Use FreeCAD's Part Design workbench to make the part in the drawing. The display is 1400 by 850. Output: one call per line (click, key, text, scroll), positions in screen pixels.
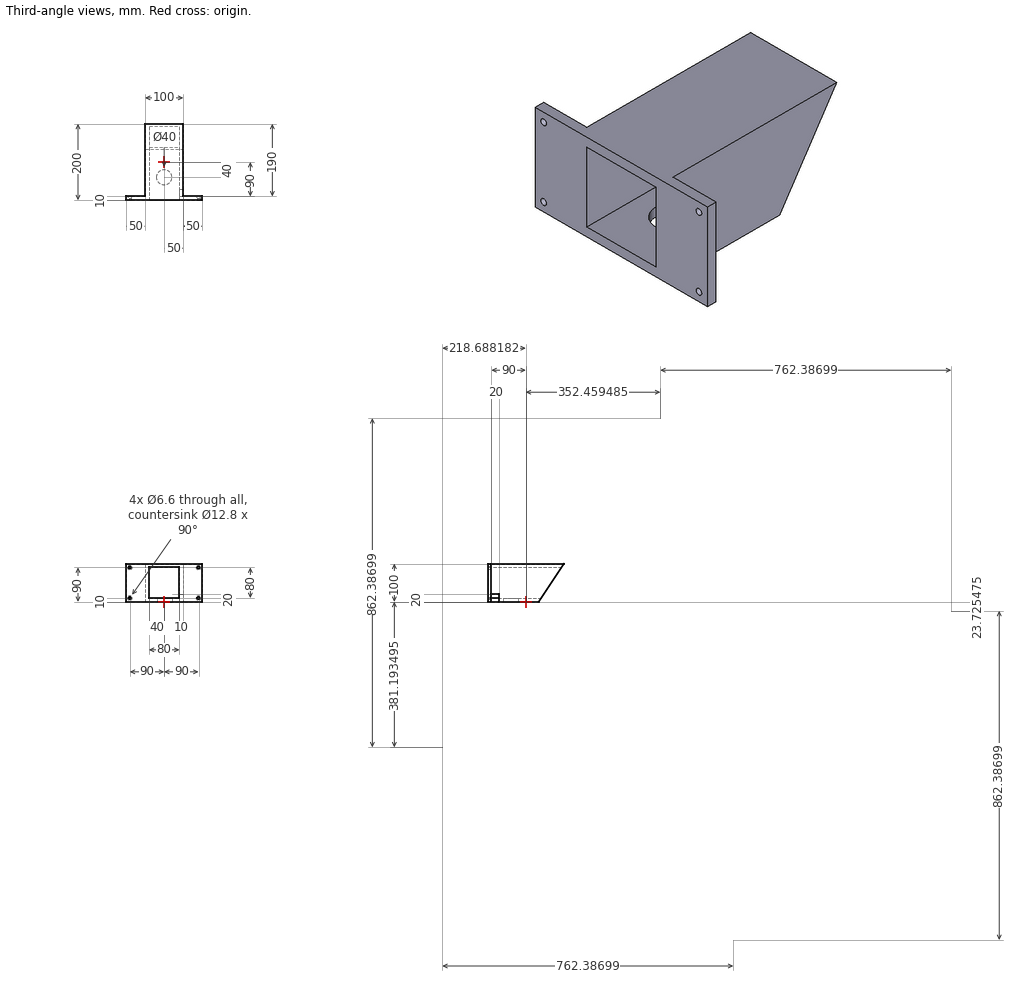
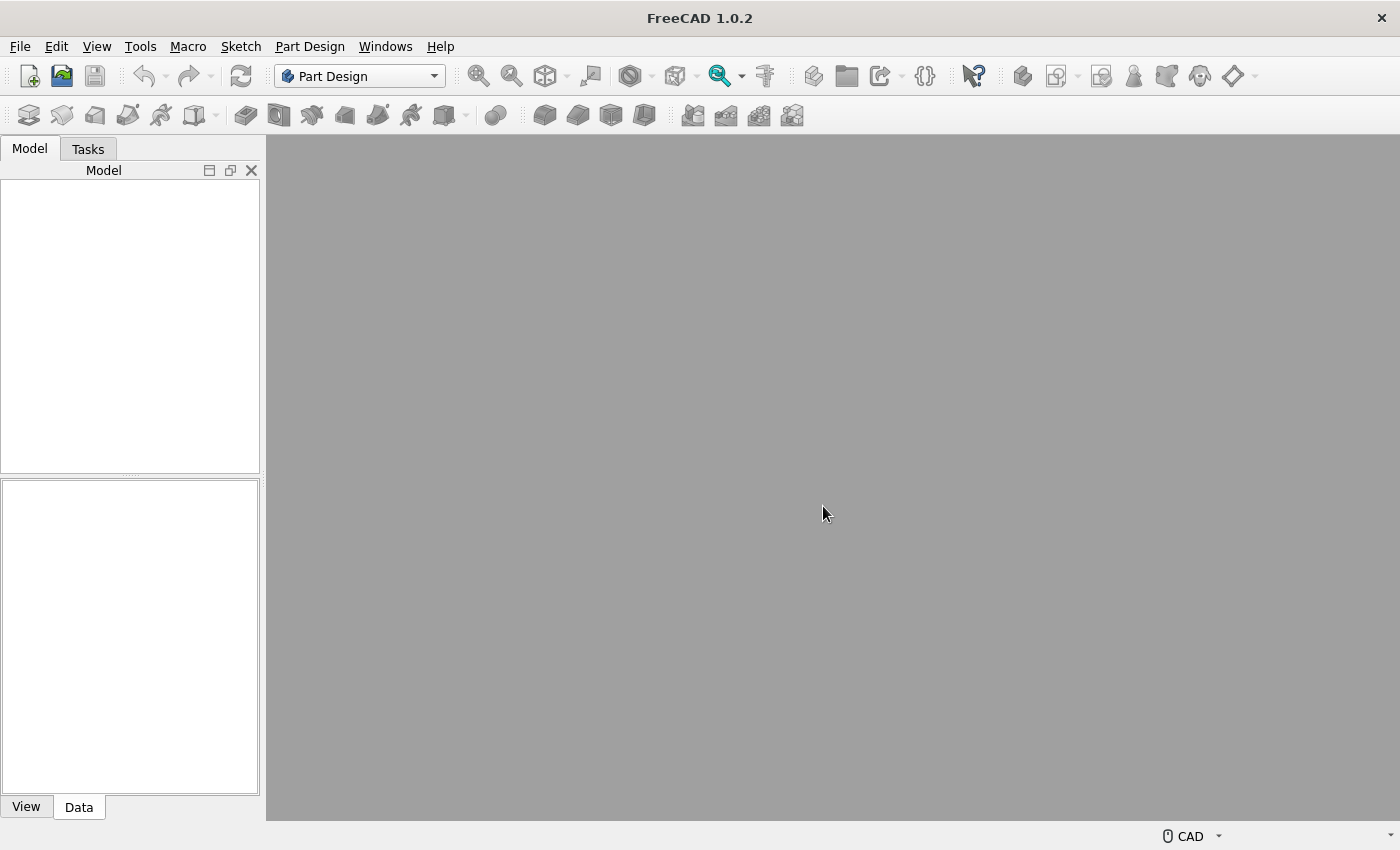
key(ctrl+n)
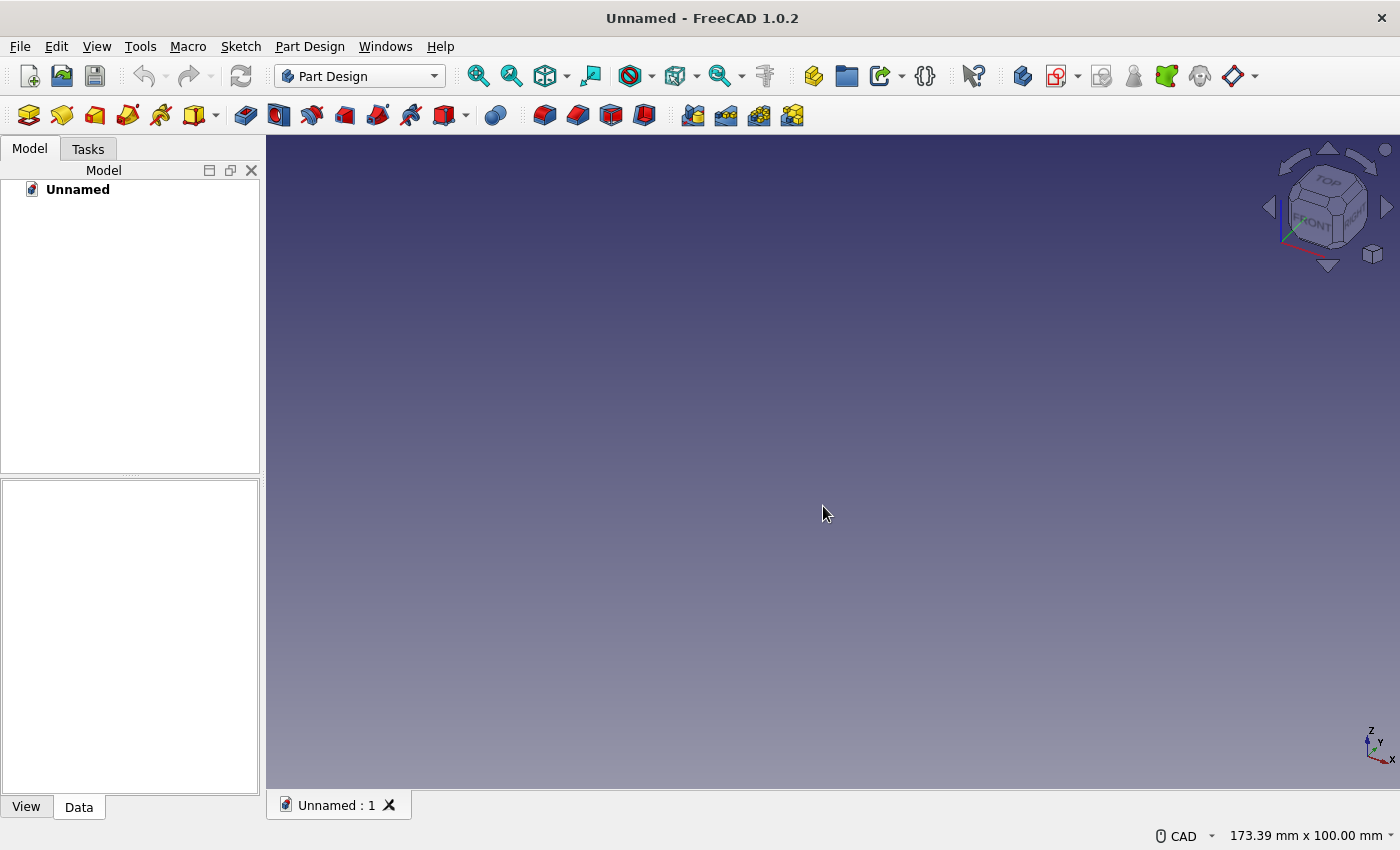
click(1056, 76)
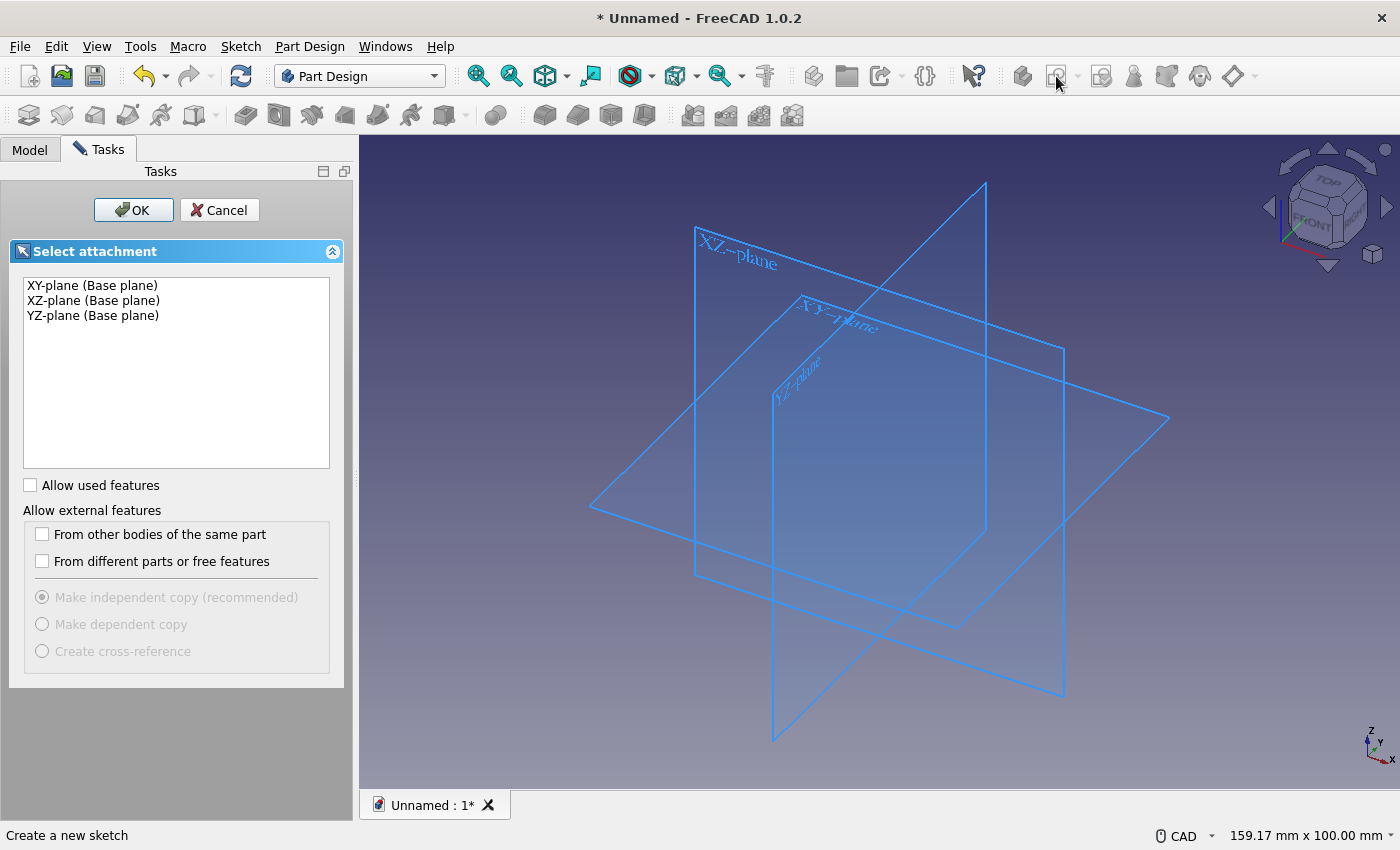
click(84, 286)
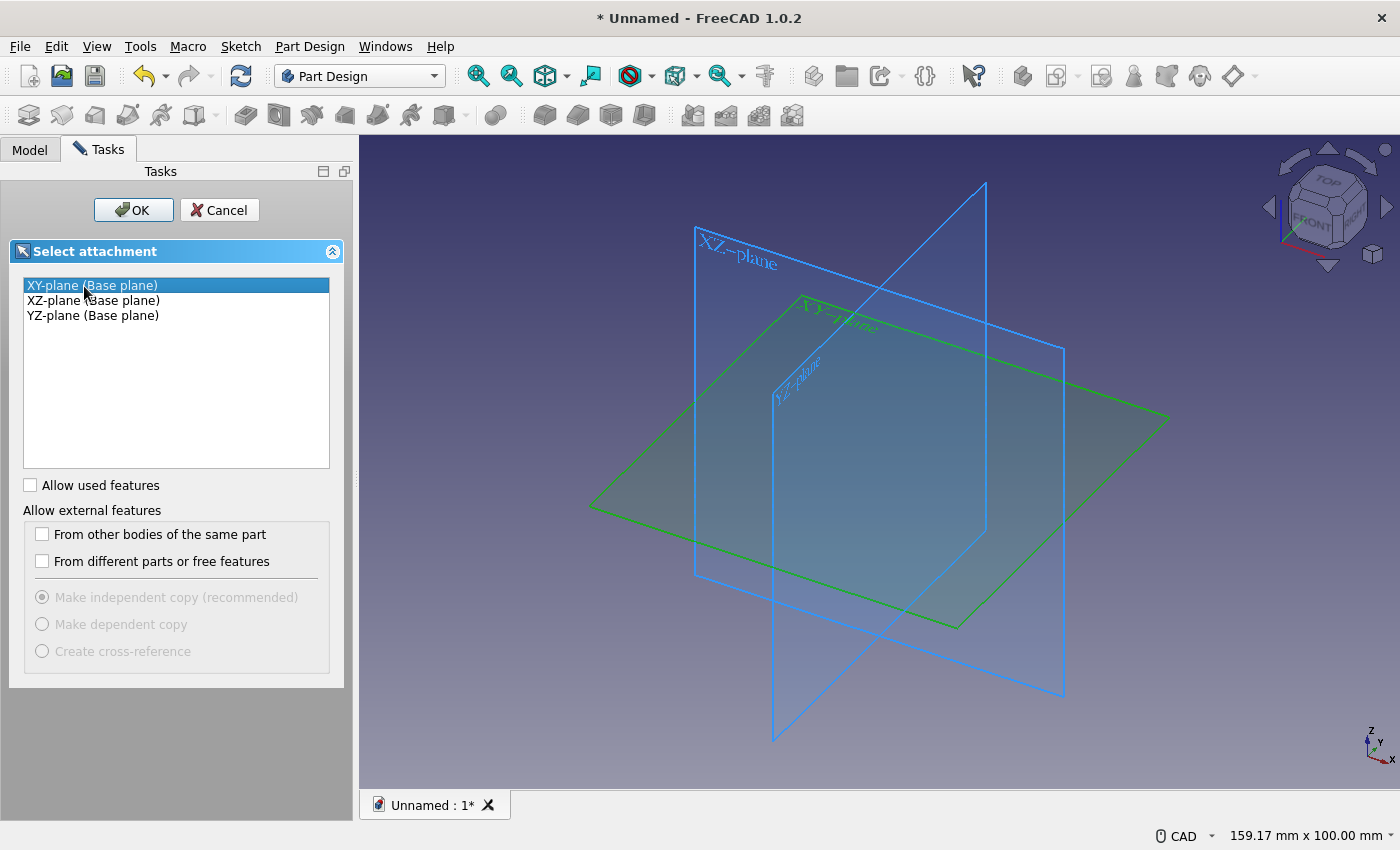
click(134, 210)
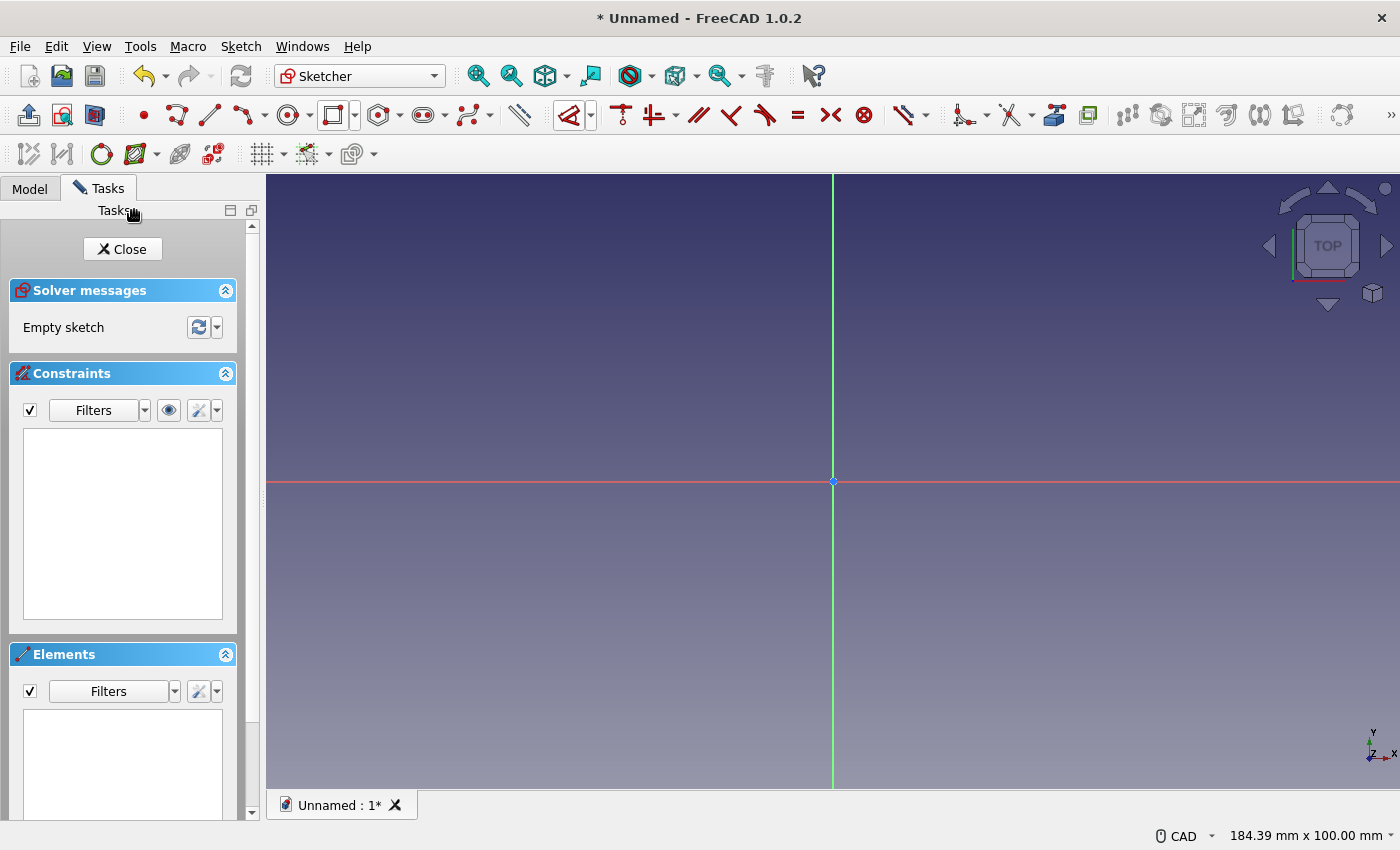
scroll(735, 482, down, 6)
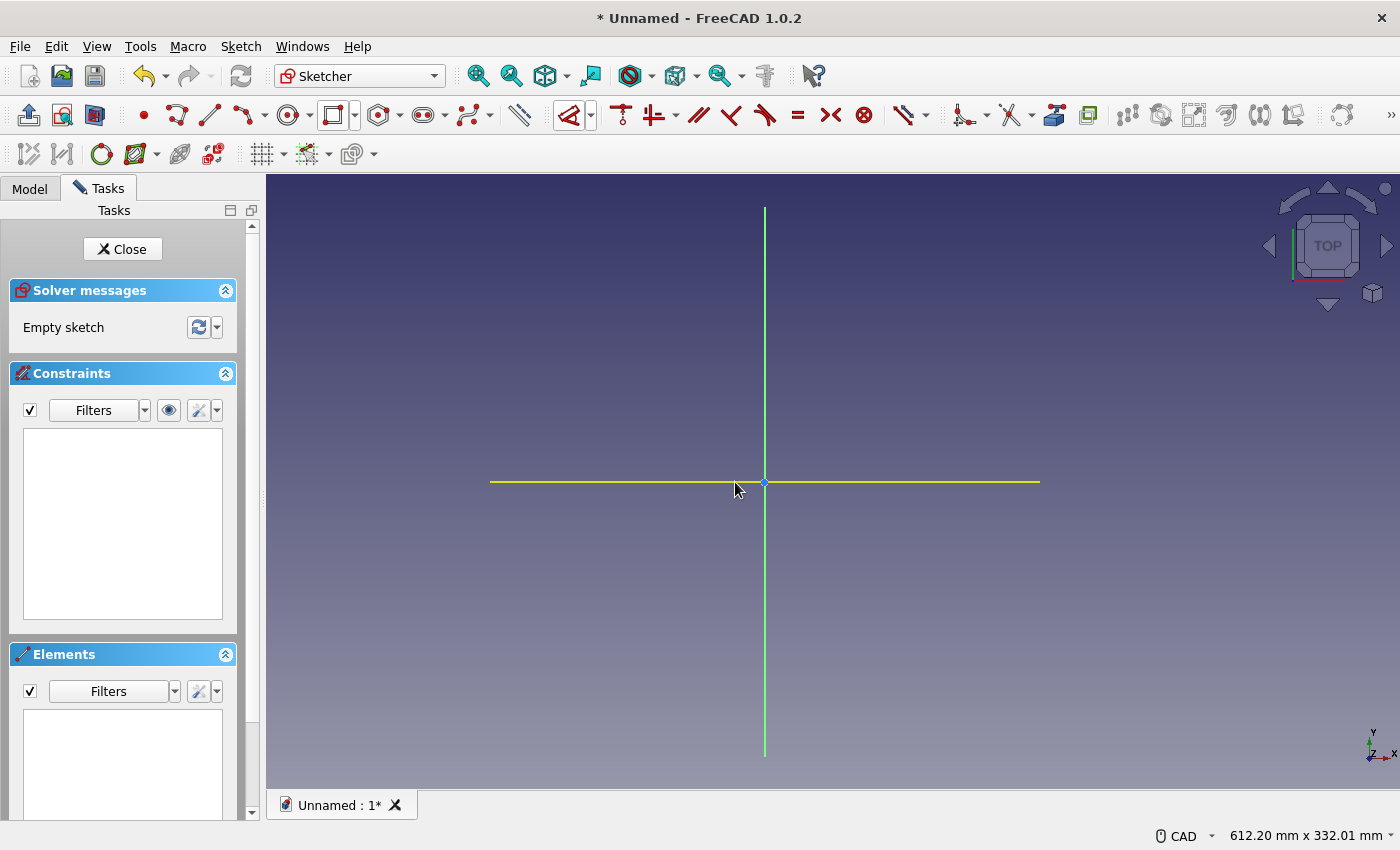
key(g)
key(m)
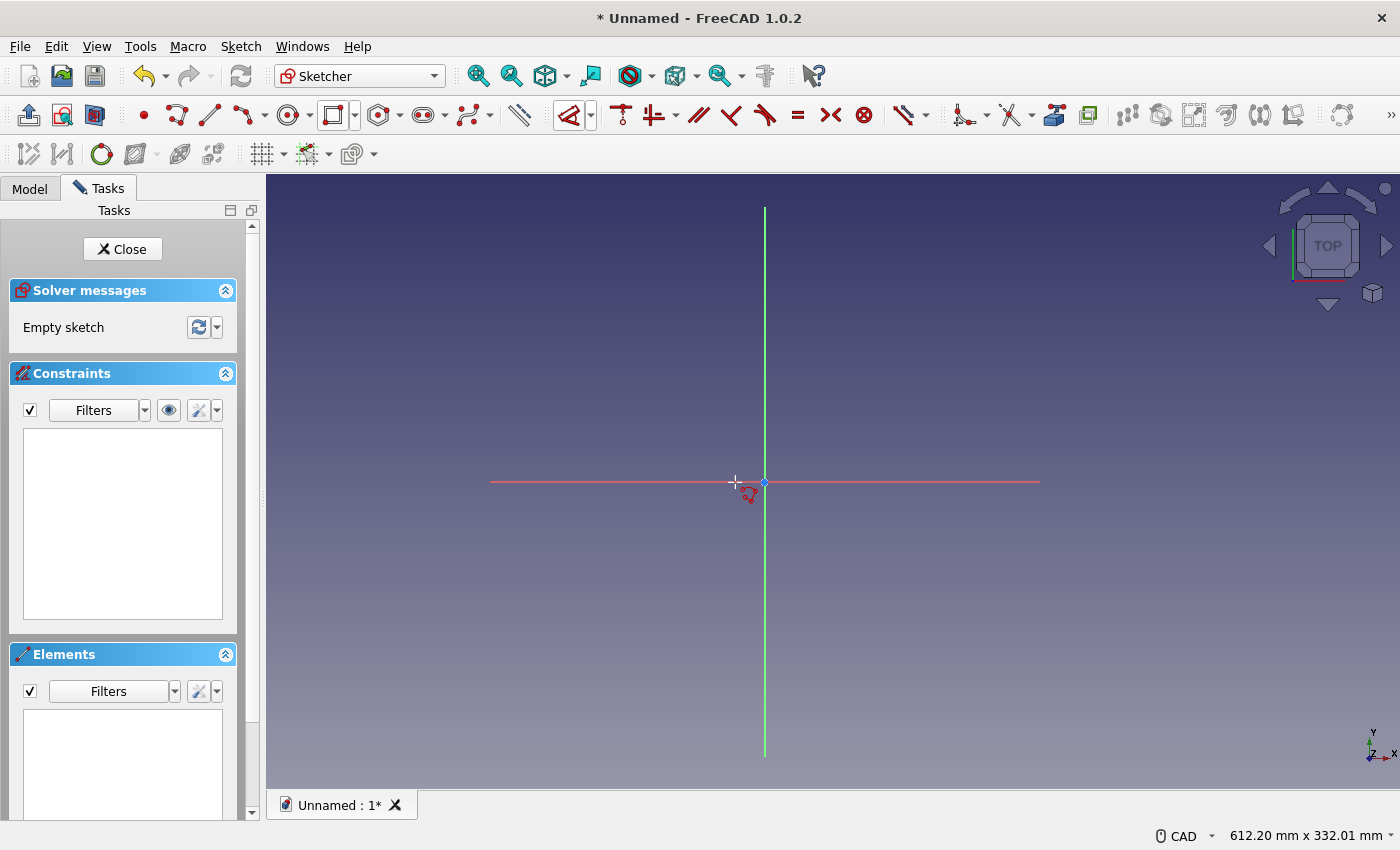
click(857, 649)
click(857, 297)
click(672, 297)
click(672, 649)
click(580, 649)
click(580, 667)
click(950, 667)
click(950, 649)
click(857, 650)
key(Escape)
key(Escape)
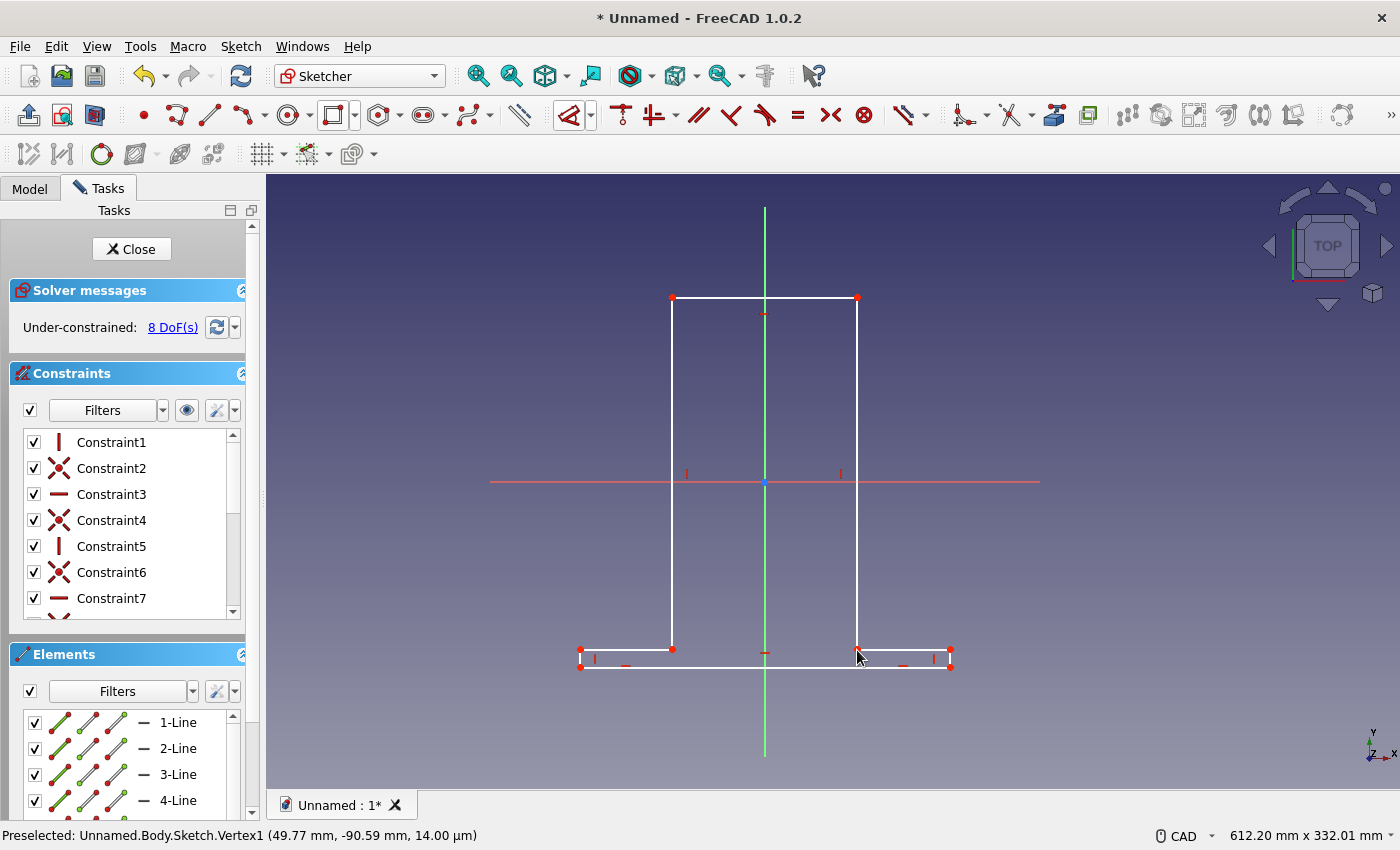
key(d)